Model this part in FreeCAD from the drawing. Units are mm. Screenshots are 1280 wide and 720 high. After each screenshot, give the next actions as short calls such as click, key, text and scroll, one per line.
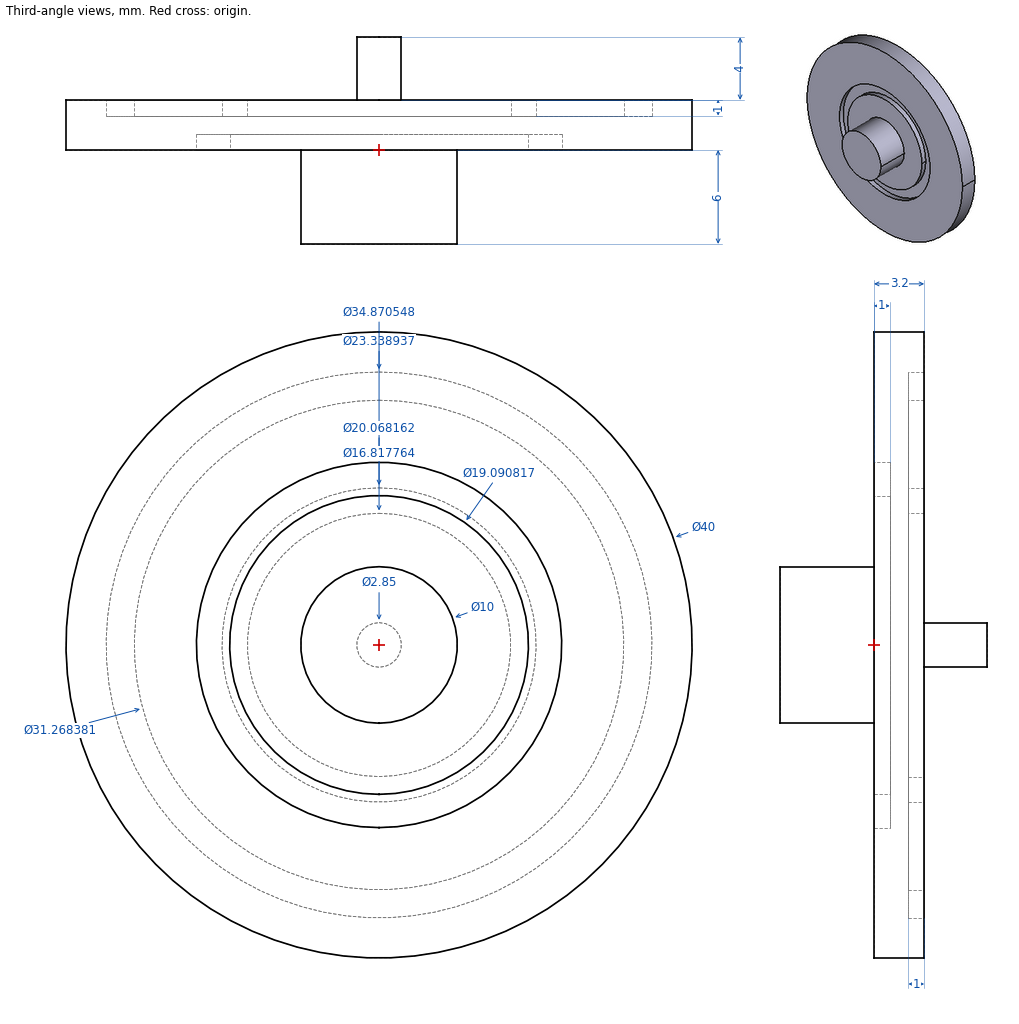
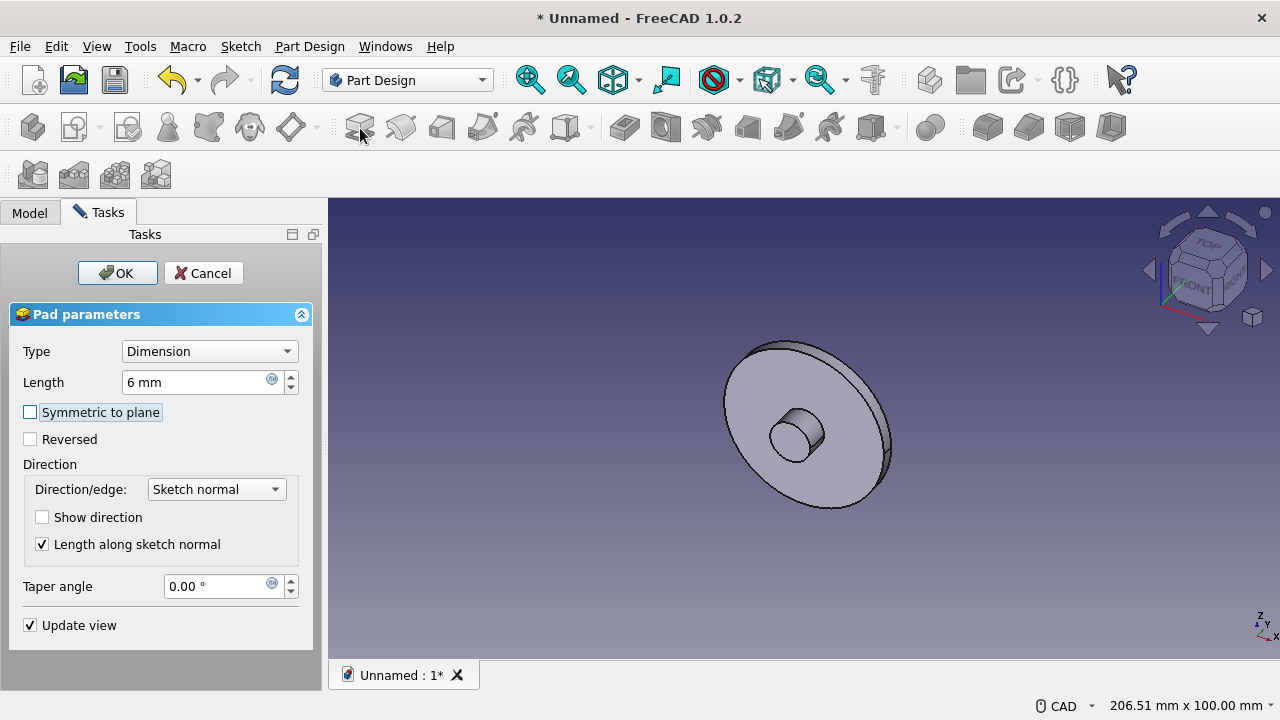
click(118, 273)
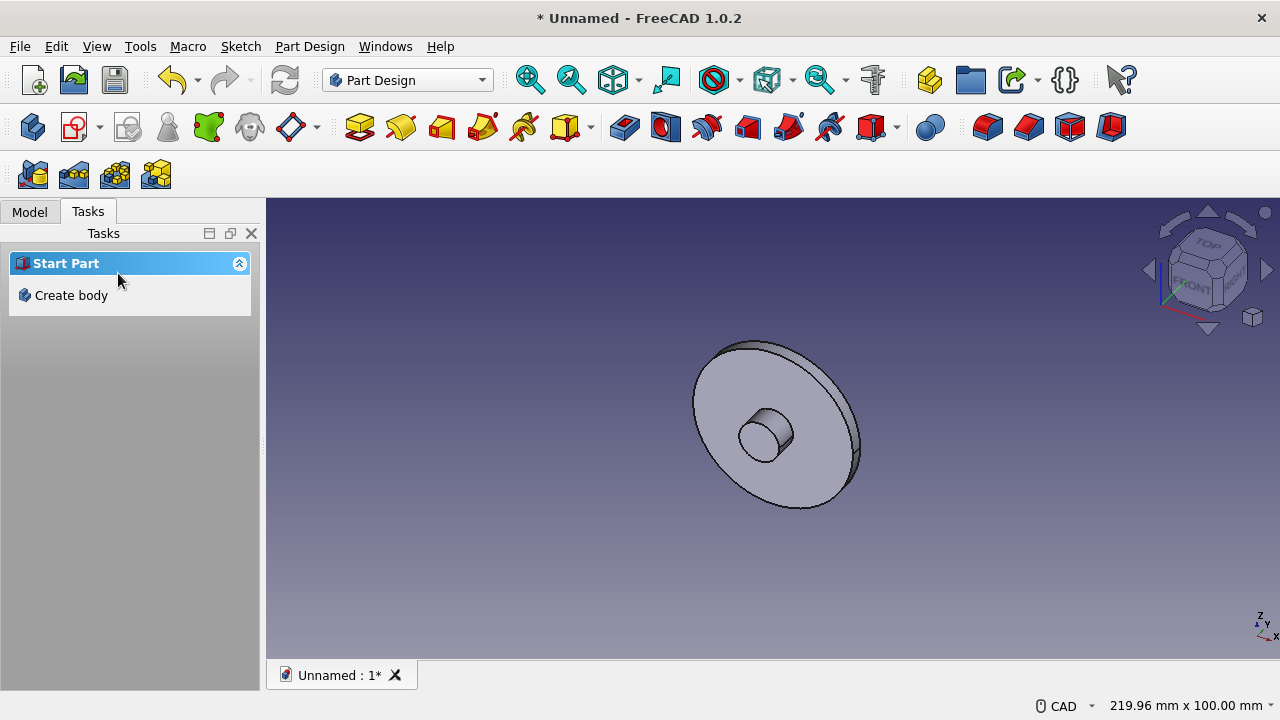
click(74, 128)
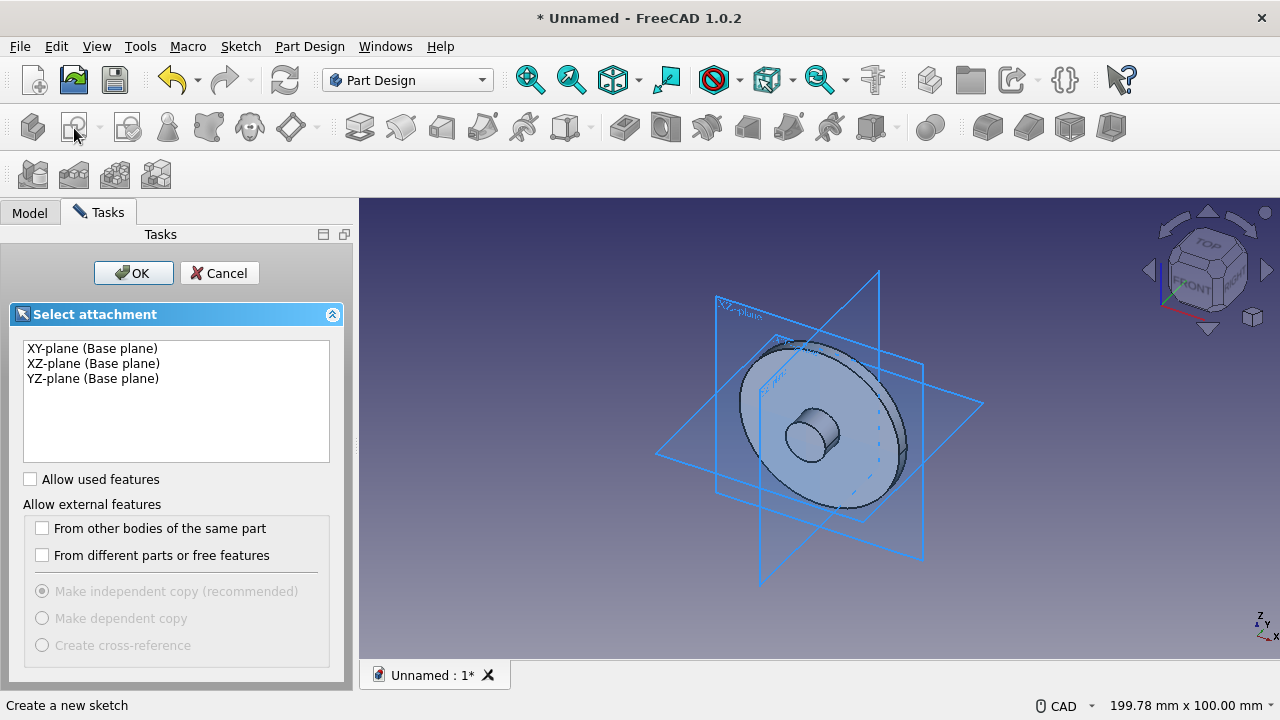
click(84, 364)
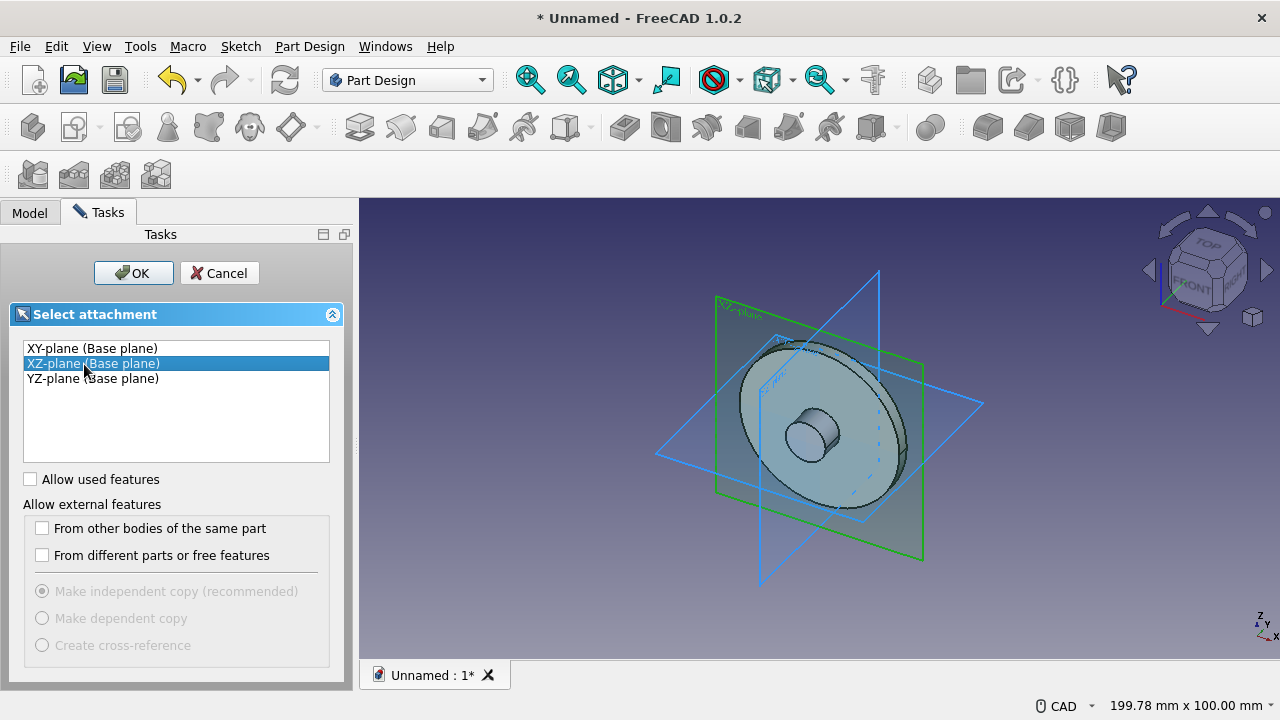
click(134, 273)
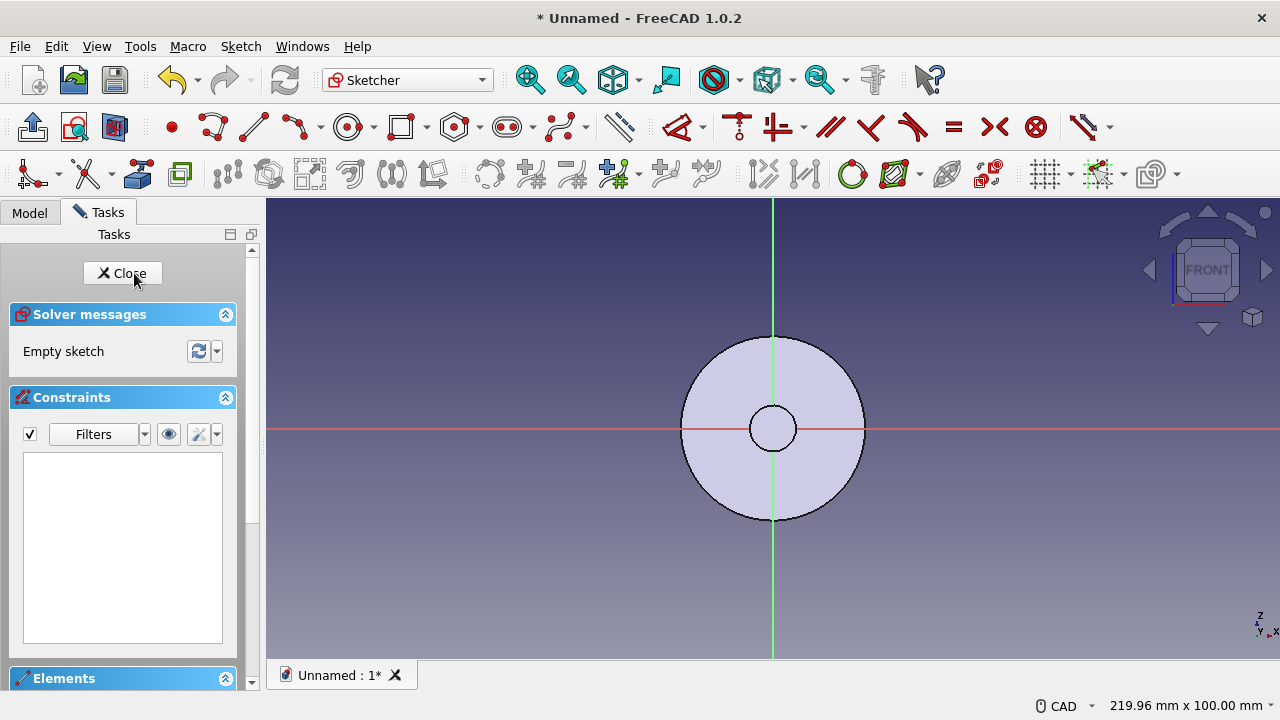
click(115, 128)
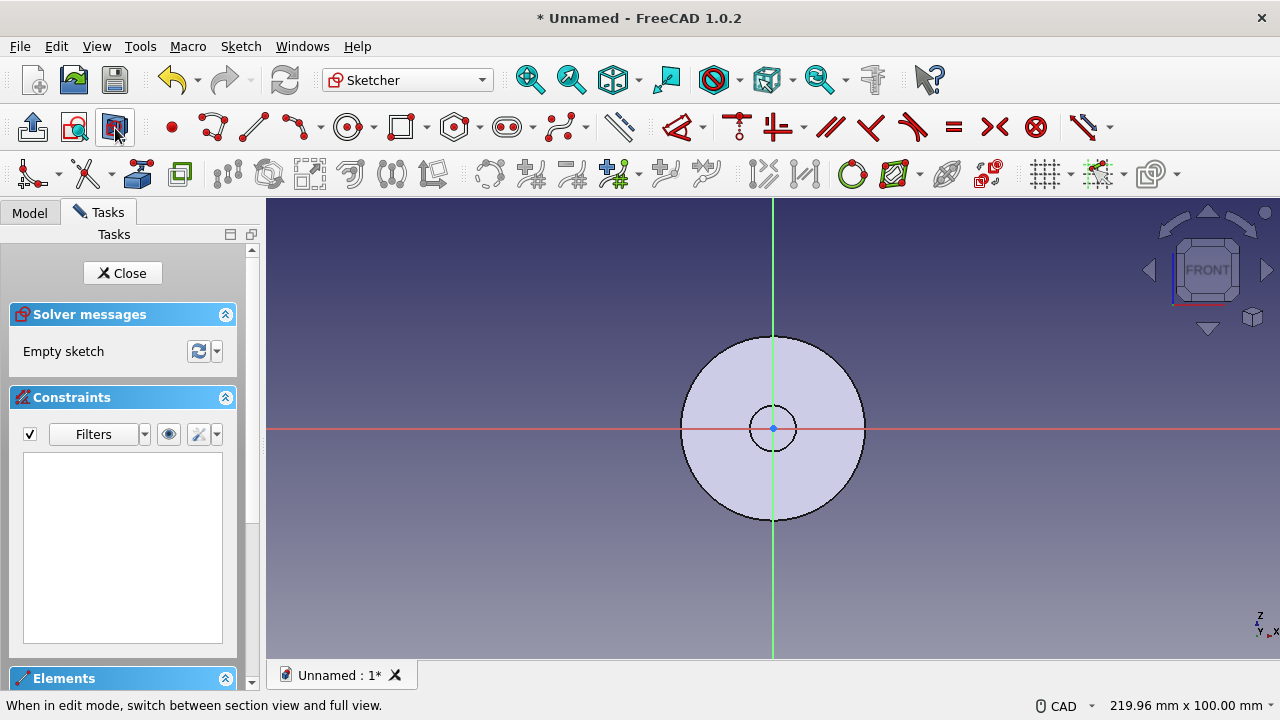
scroll(813, 429, up, 5)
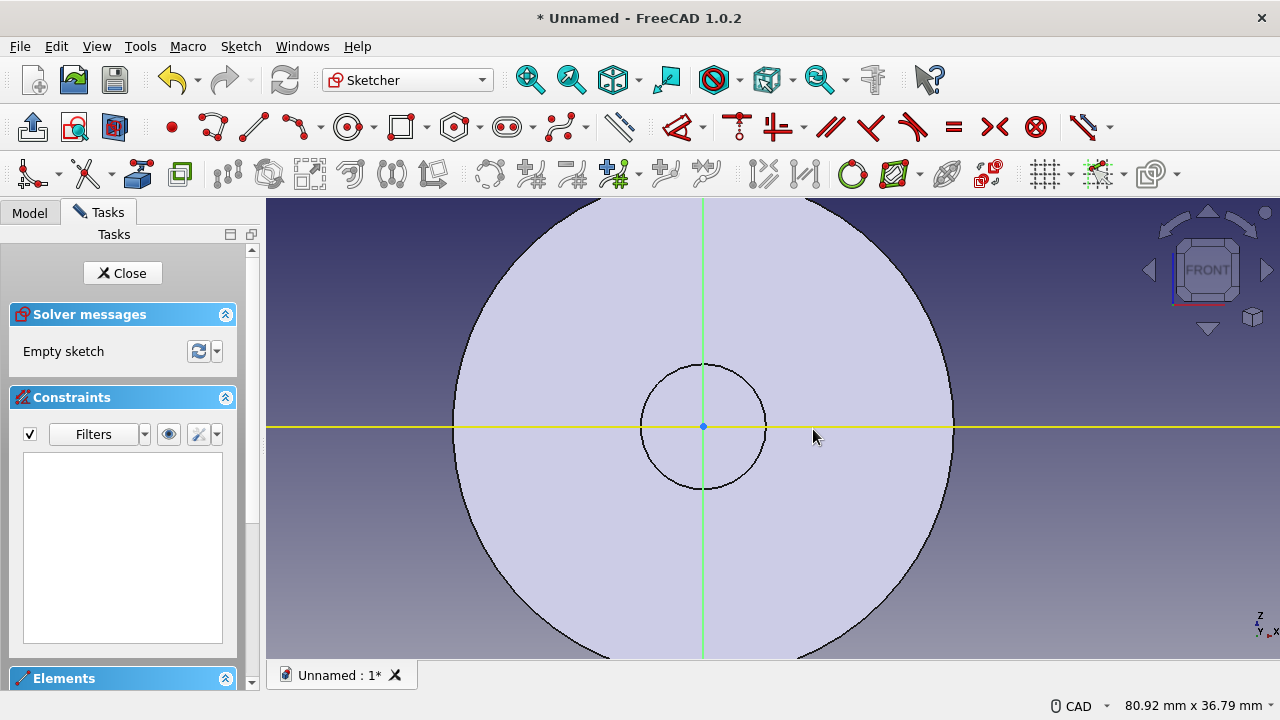
click(348, 128)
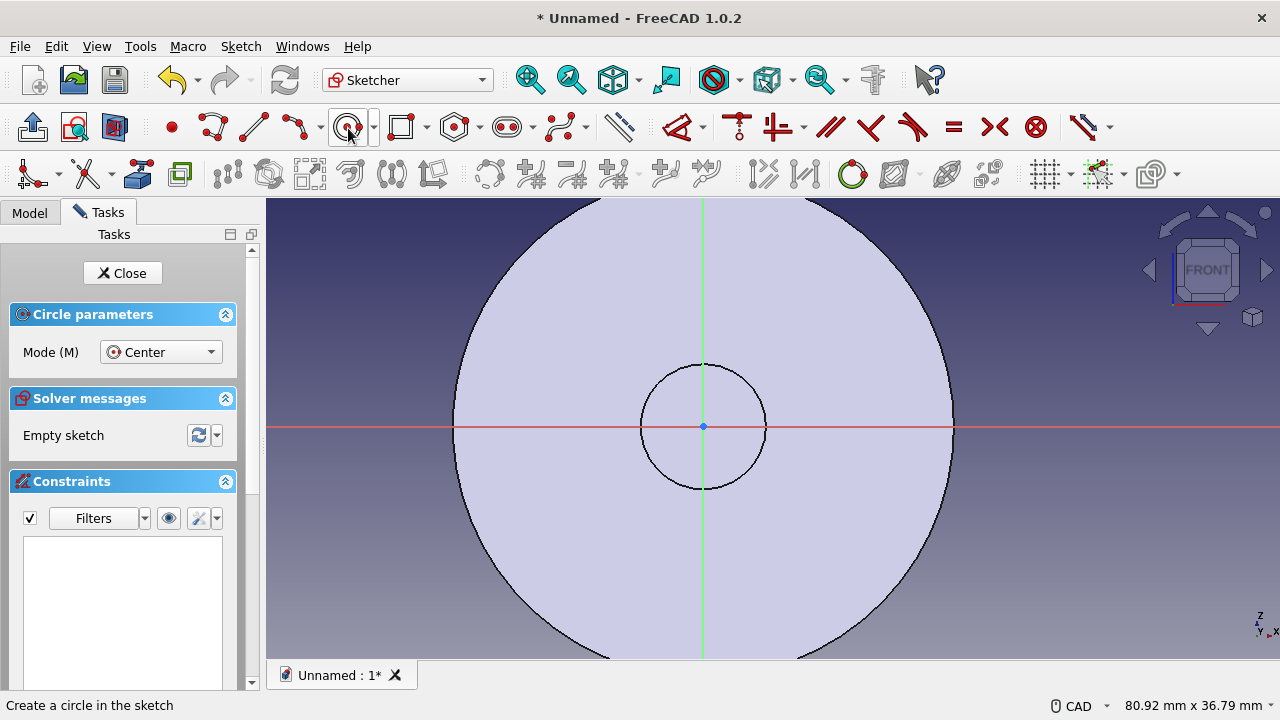
click(703, 427)
move(807, 323)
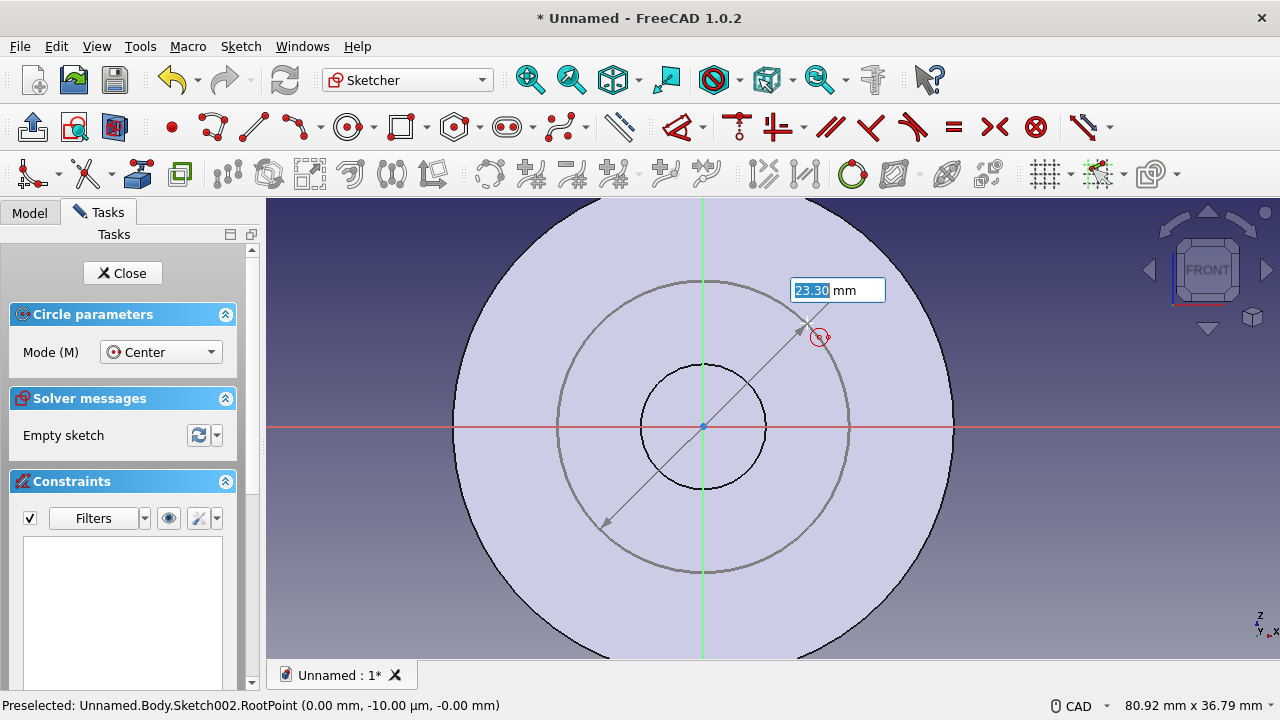
text(23.338937)
key(Return)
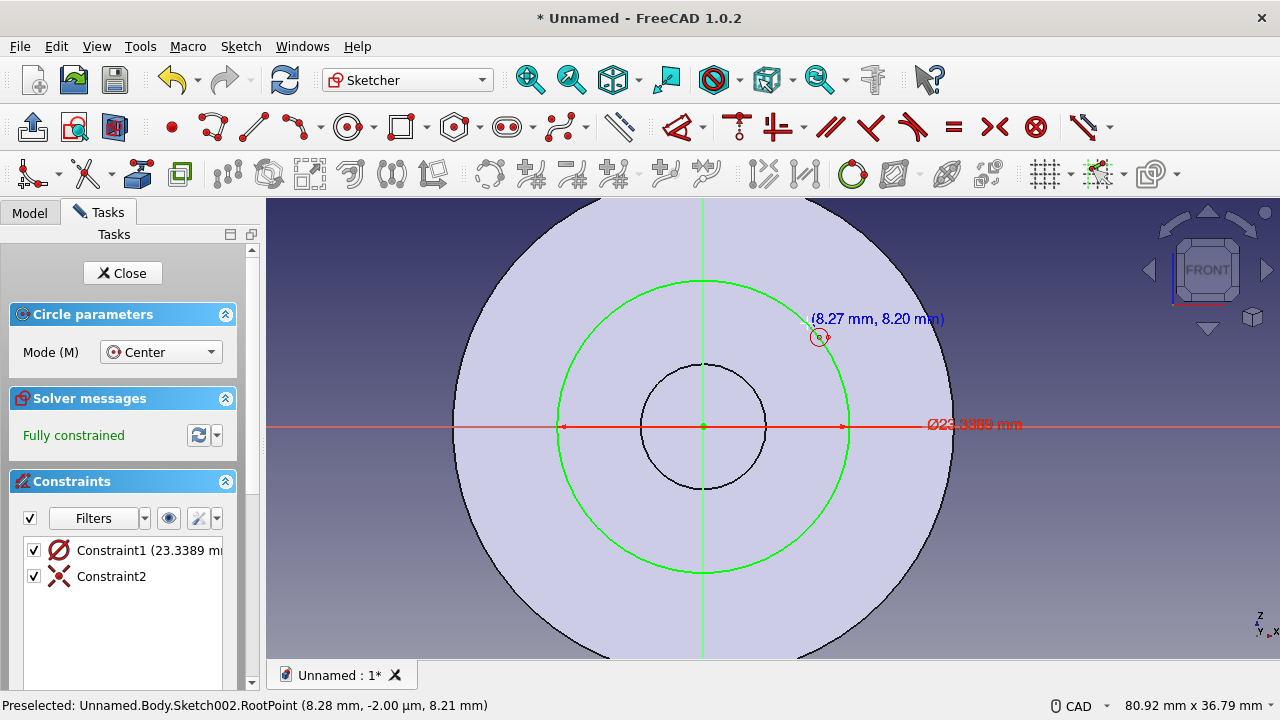
click(703, 427)
move(788, 342)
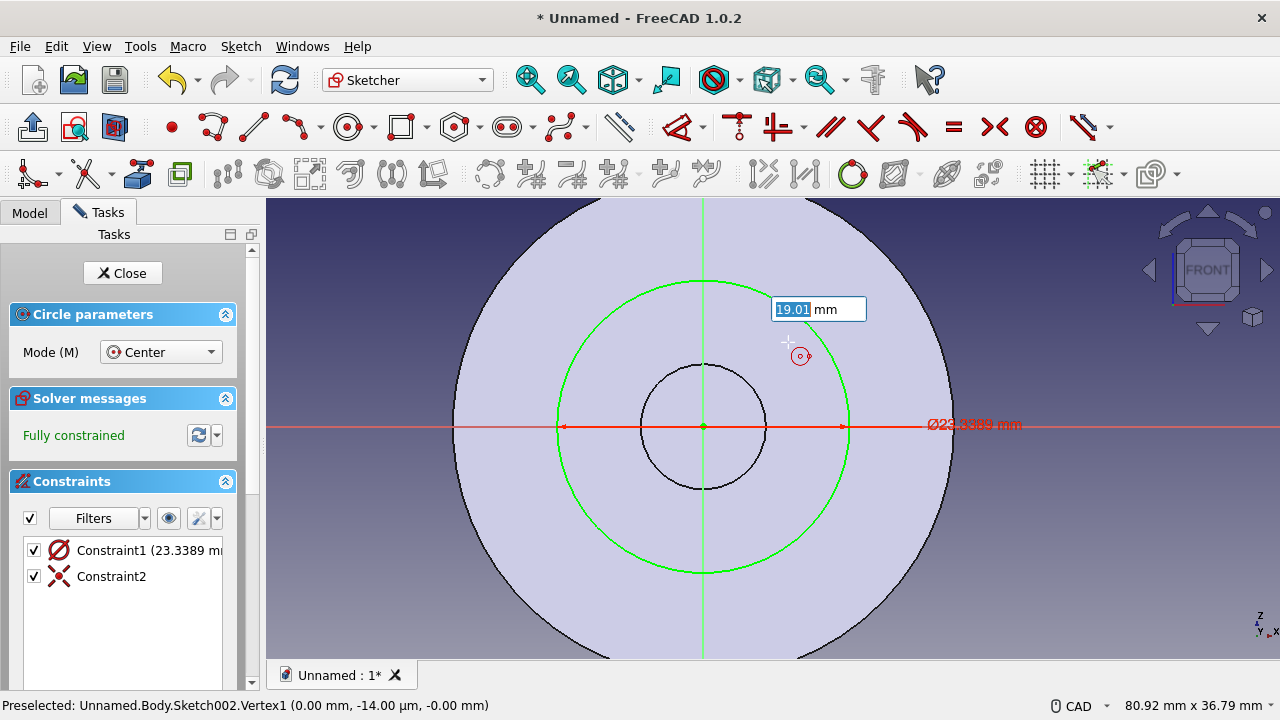
text(19.090817)
key(Return)
key(Escape)